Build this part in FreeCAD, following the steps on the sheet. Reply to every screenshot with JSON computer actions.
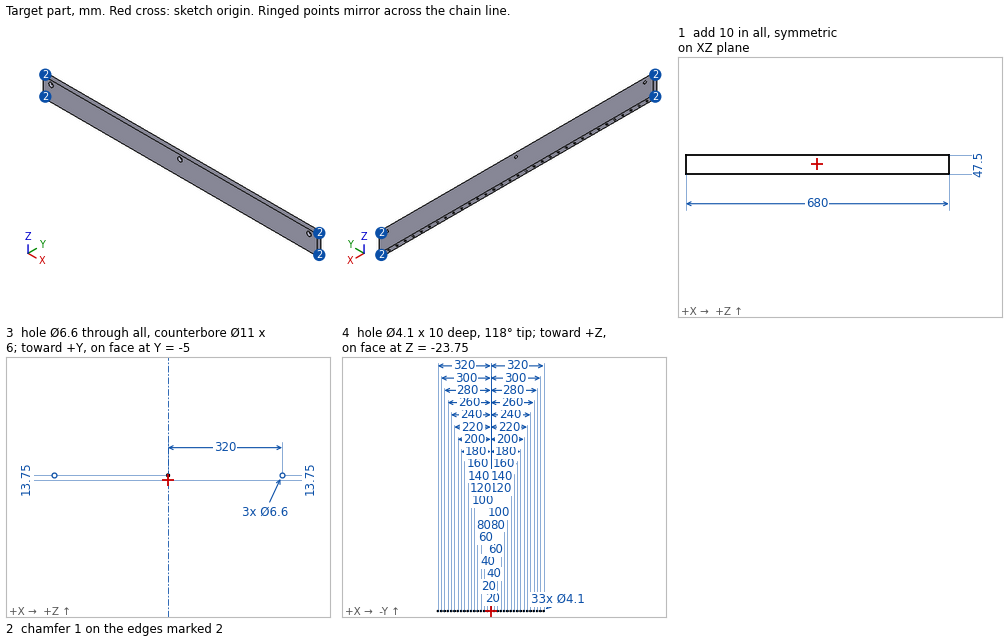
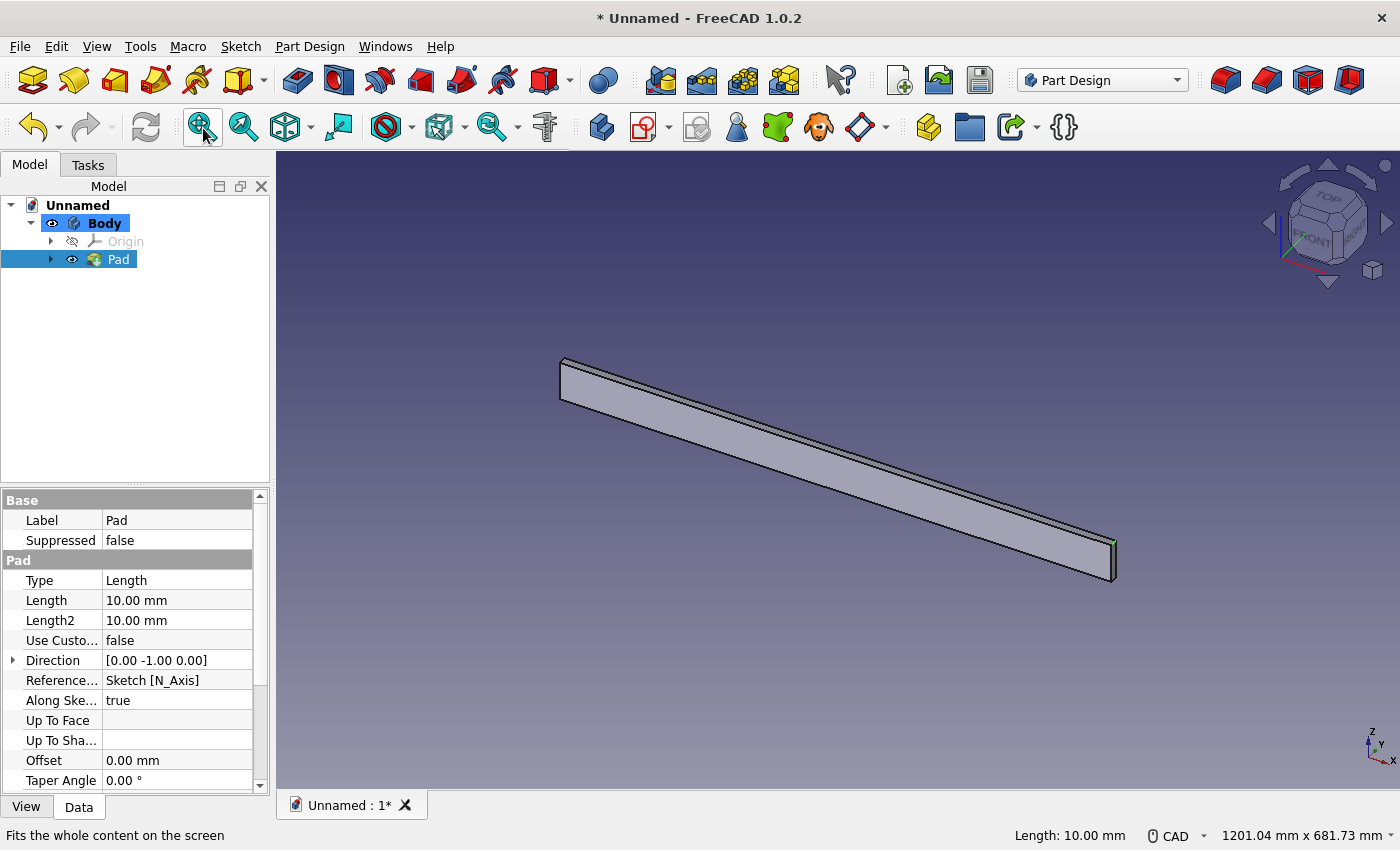
{"action": "key", "text": "0"}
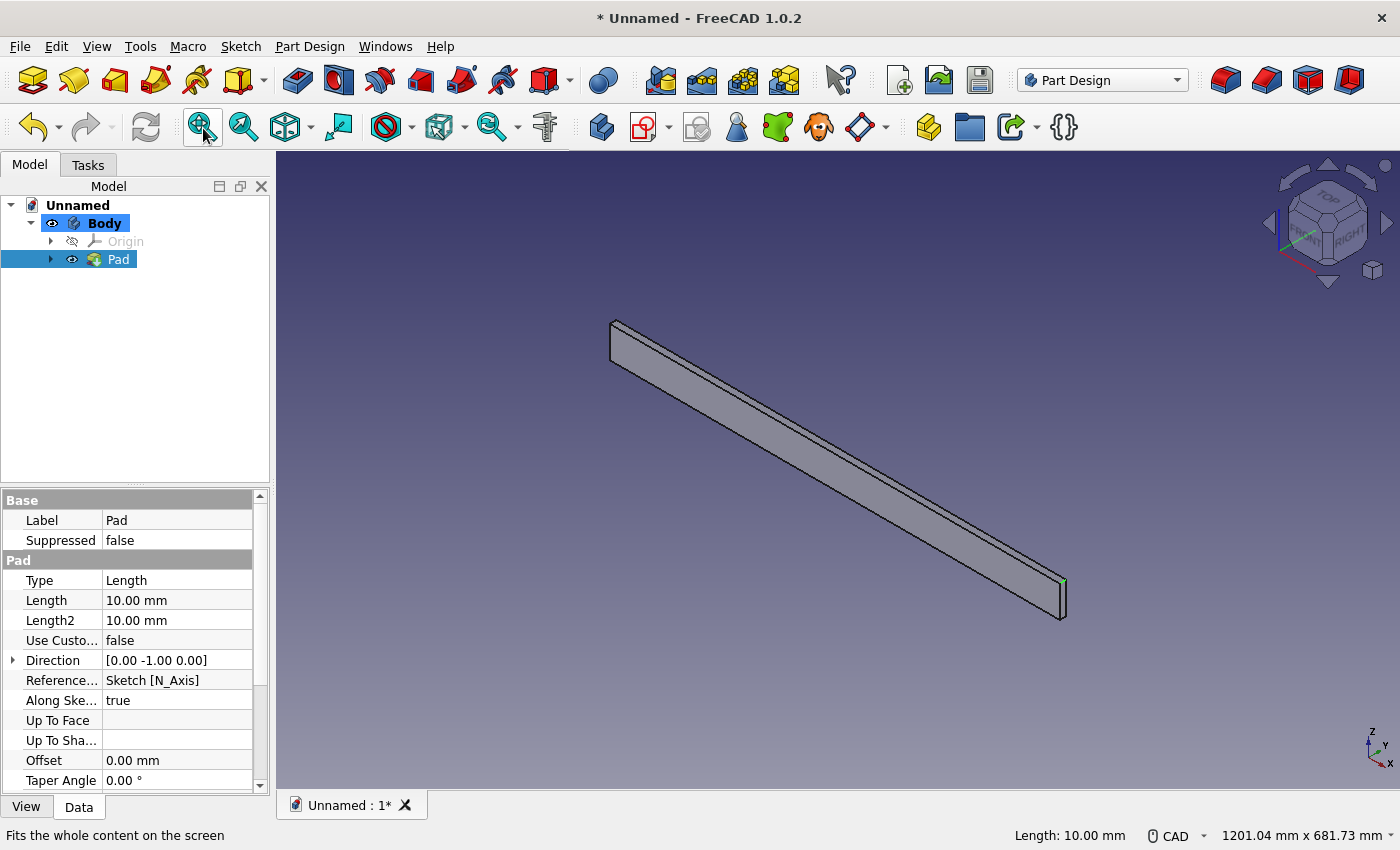
{"action": "scroll", "coordinate": [613, 321], "scroll_direction": "up", "scroll_amount": 8}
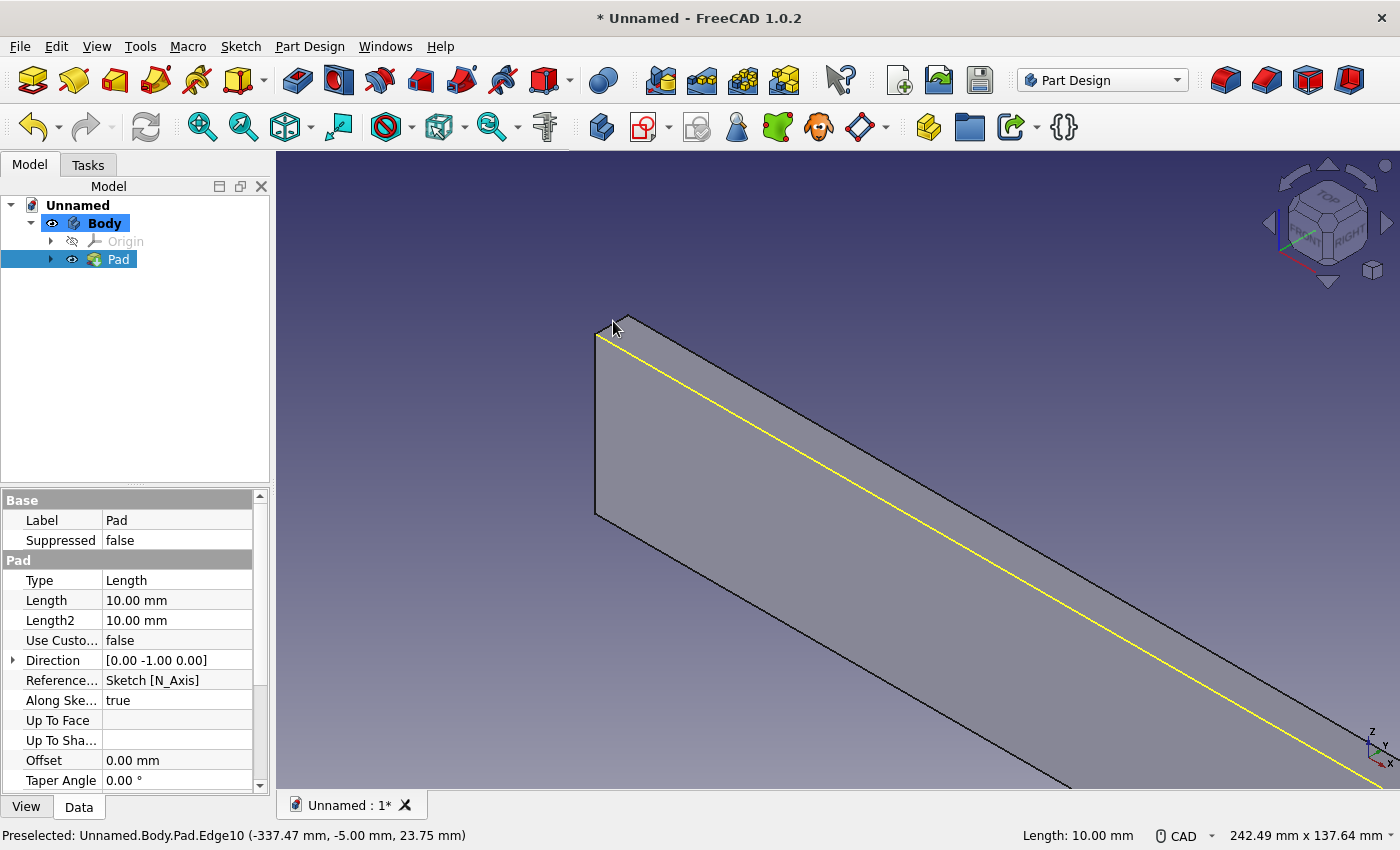
{"action": "left_click", "coordinate": [203, 128]}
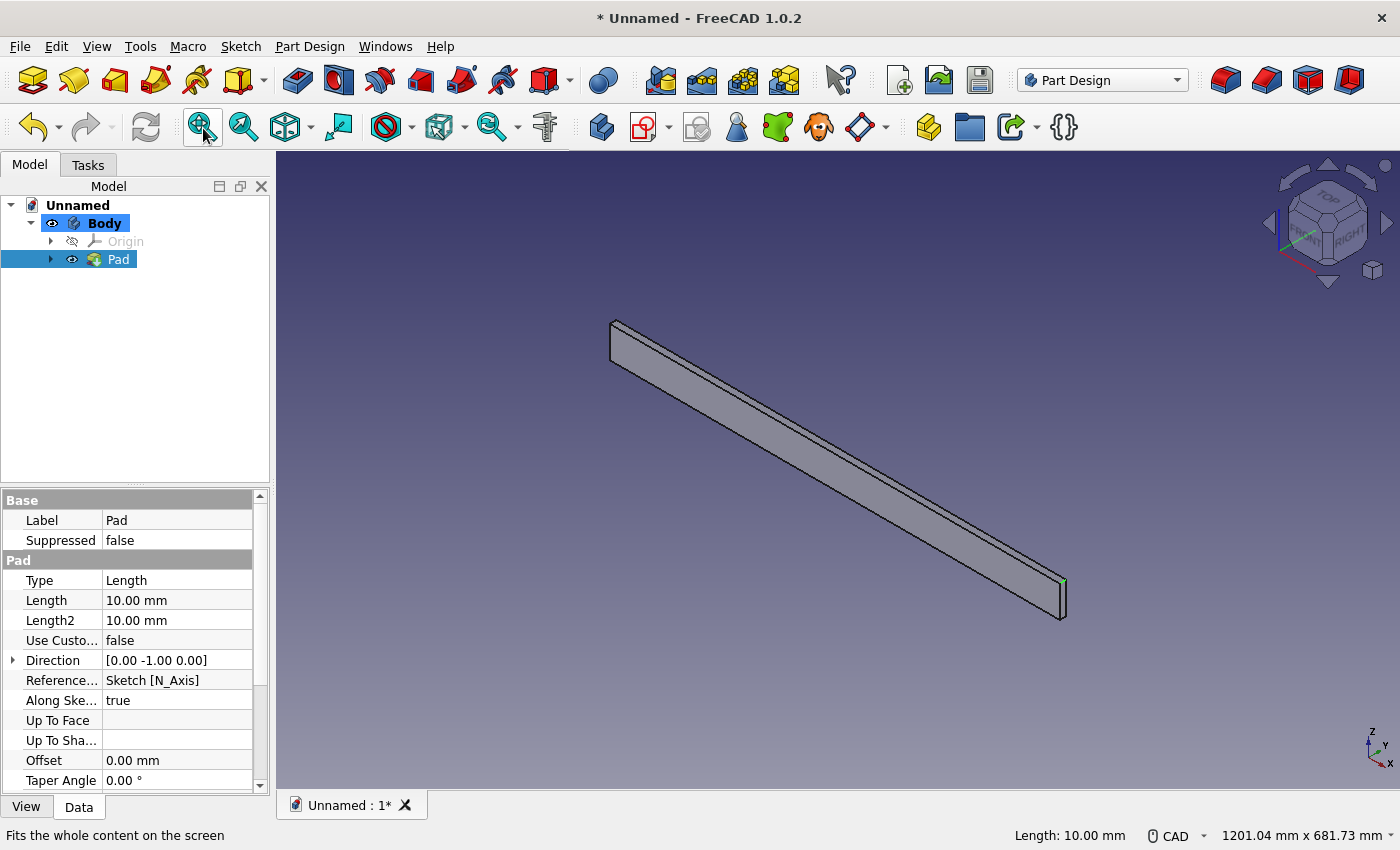
{"action": "key", "text": "2"}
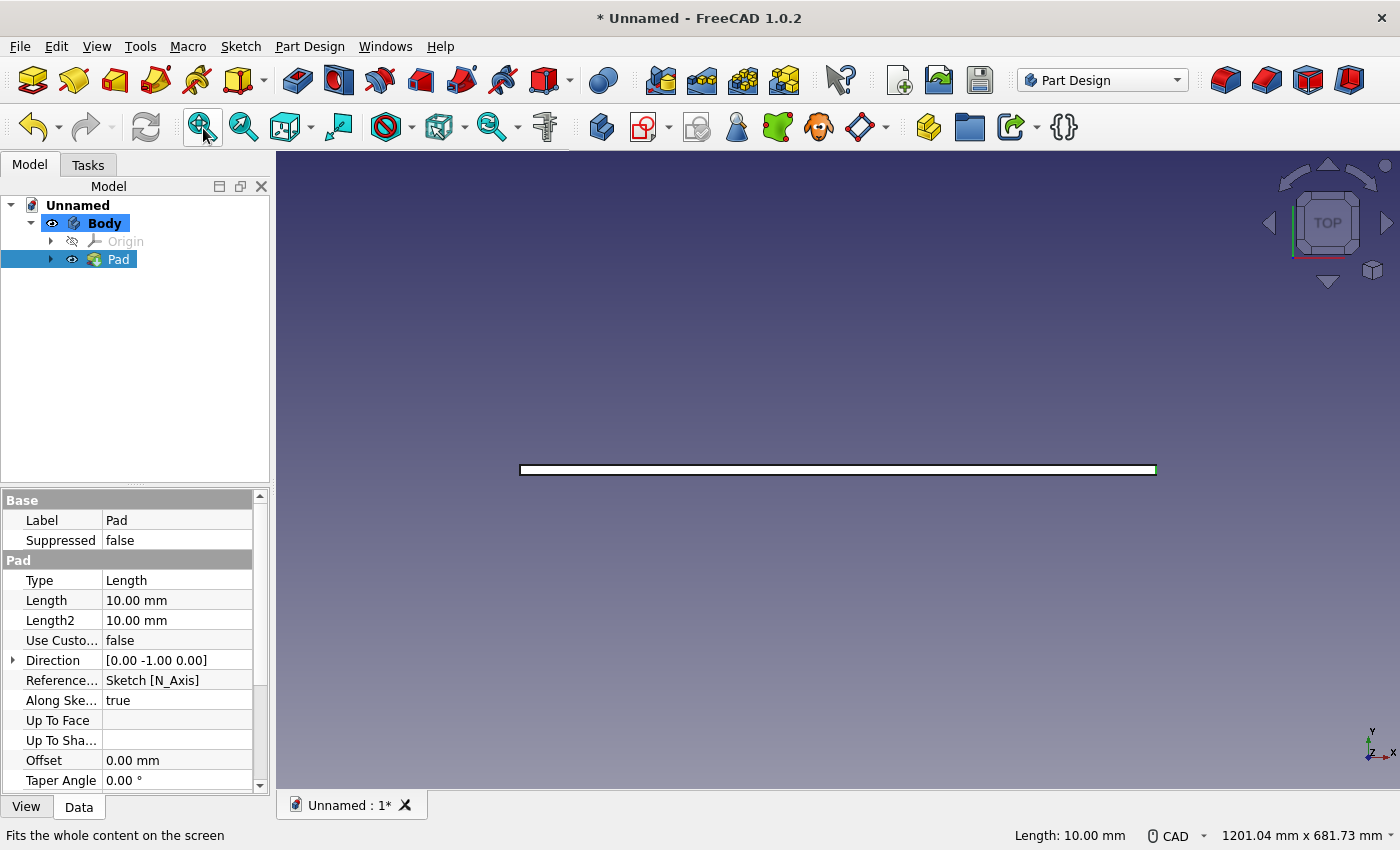
{"action": "left_click", "coordinate": [520, 471], "text": "ctrl"}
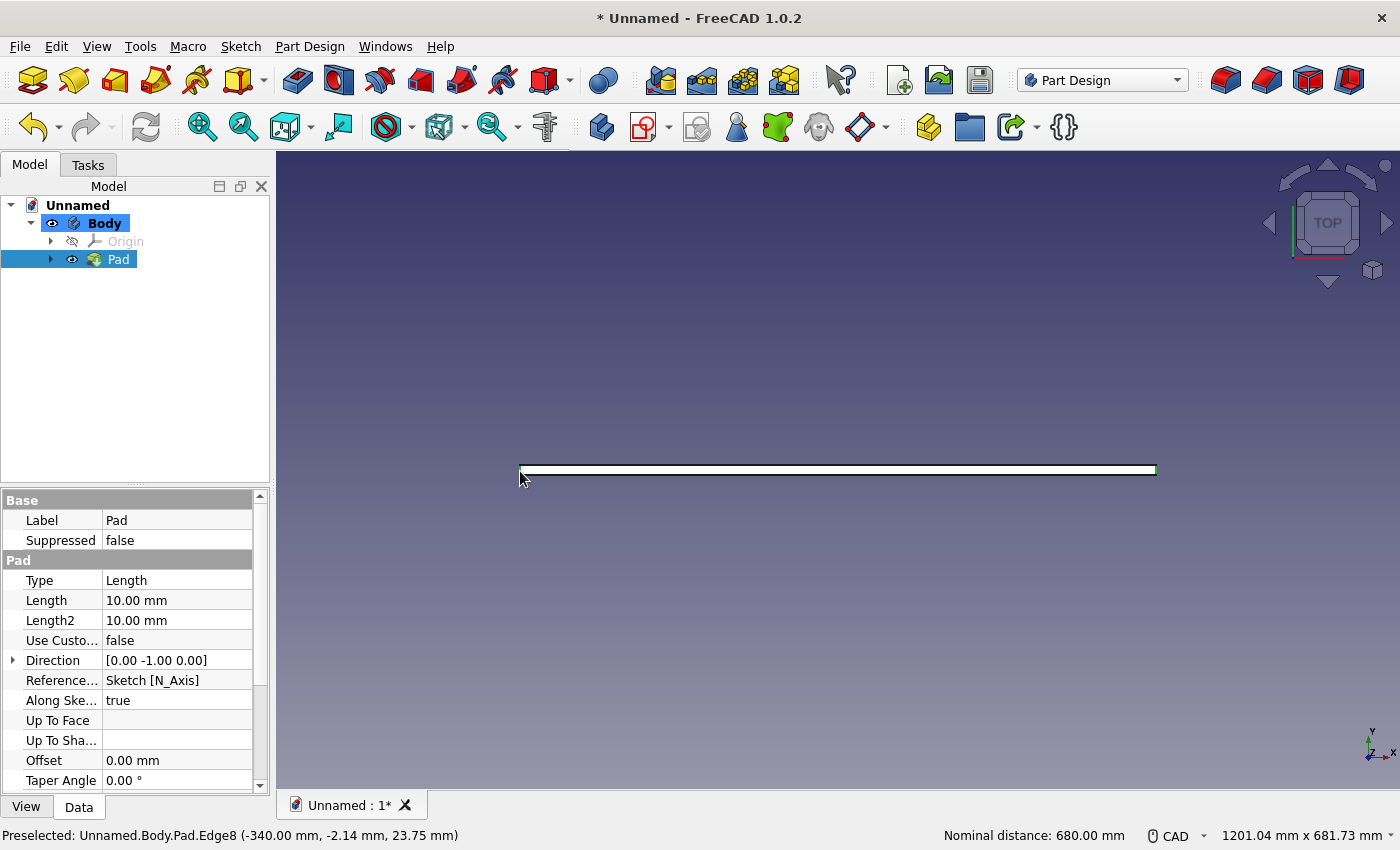
{"action": "scroll", "coordinate": [520, 469], "scroll_direction": "up", "scroll_amount": 8}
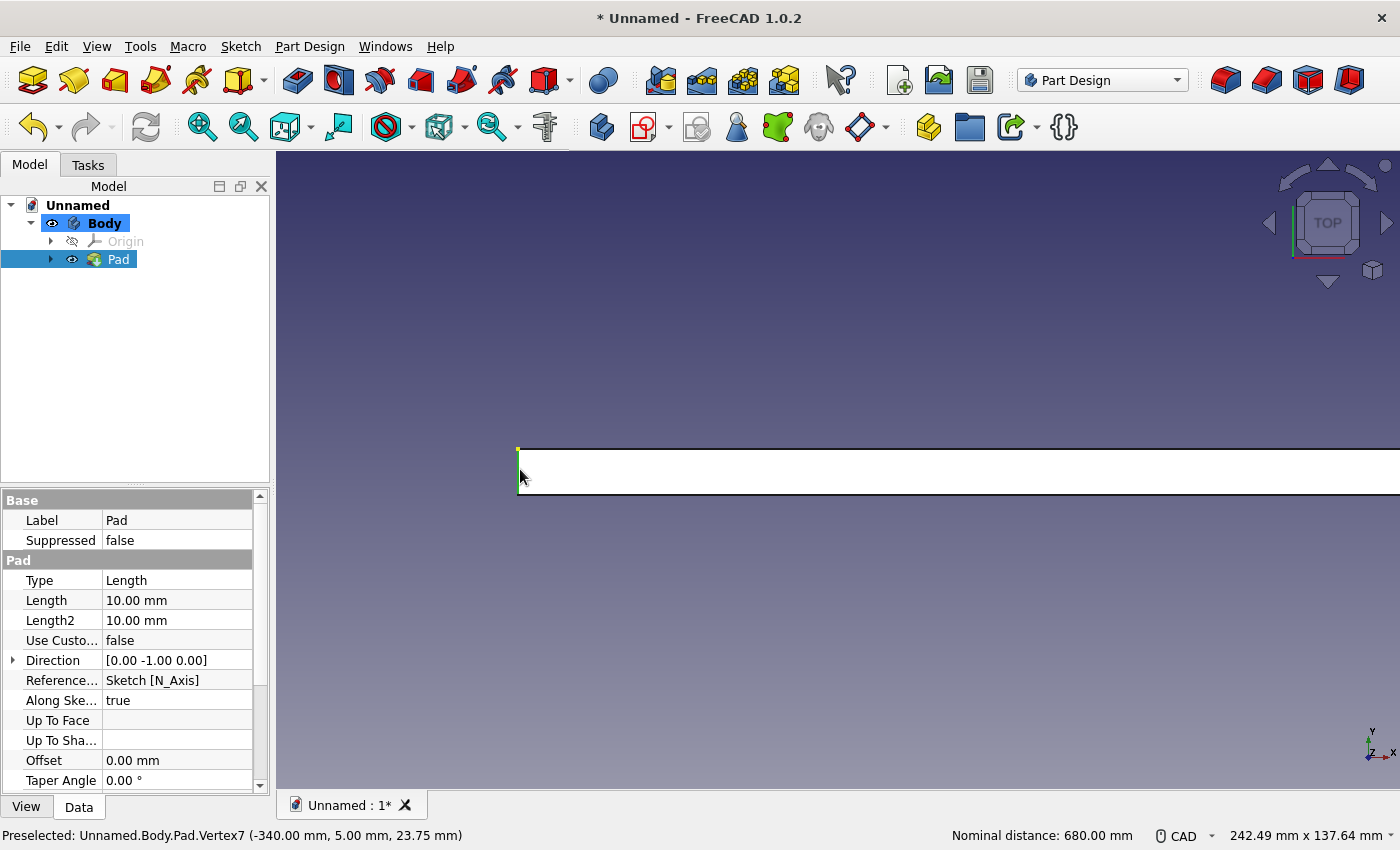
{"action": "left_click", "coordinate": [203, 128]}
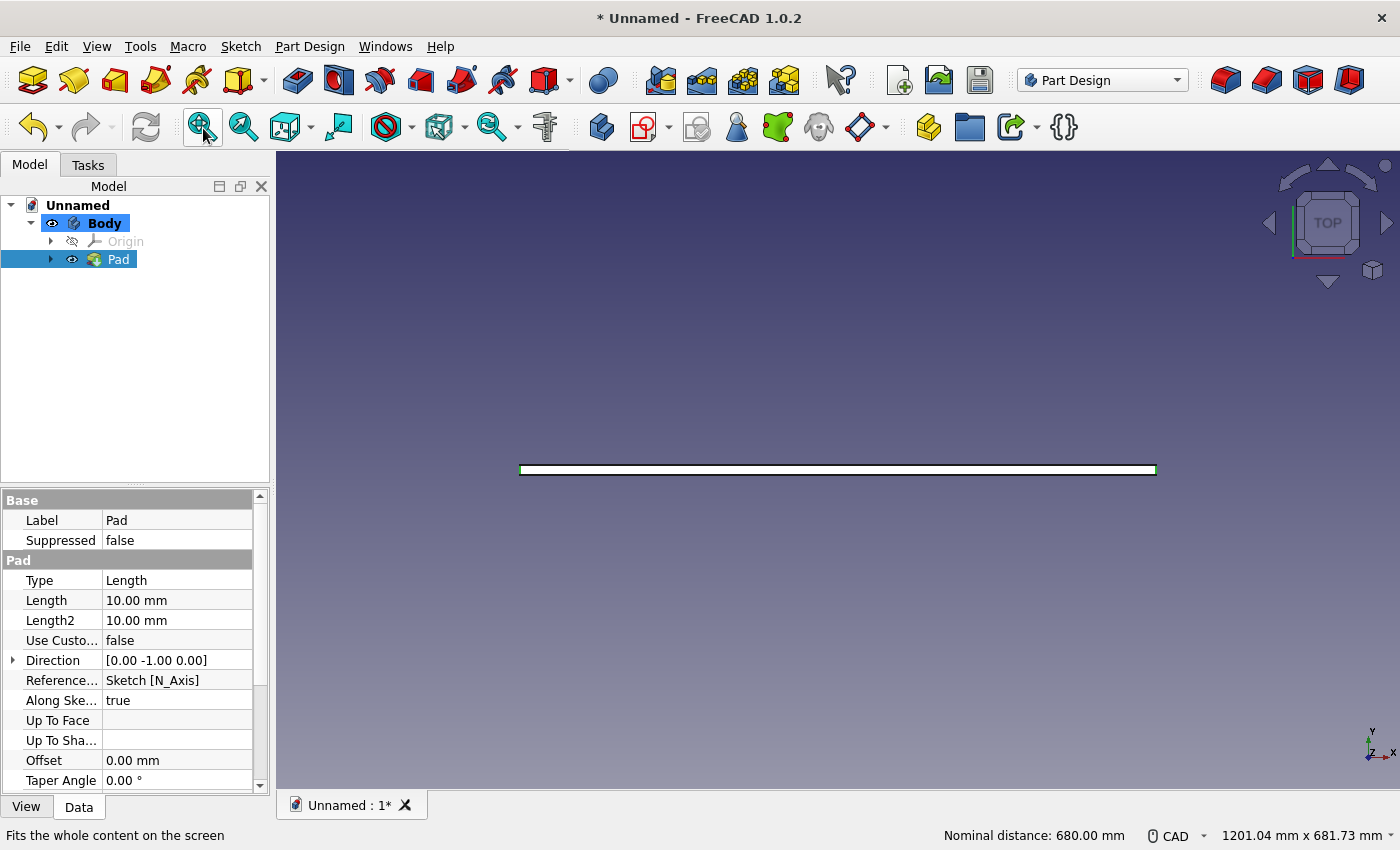
{"action": "key", "text": "1"}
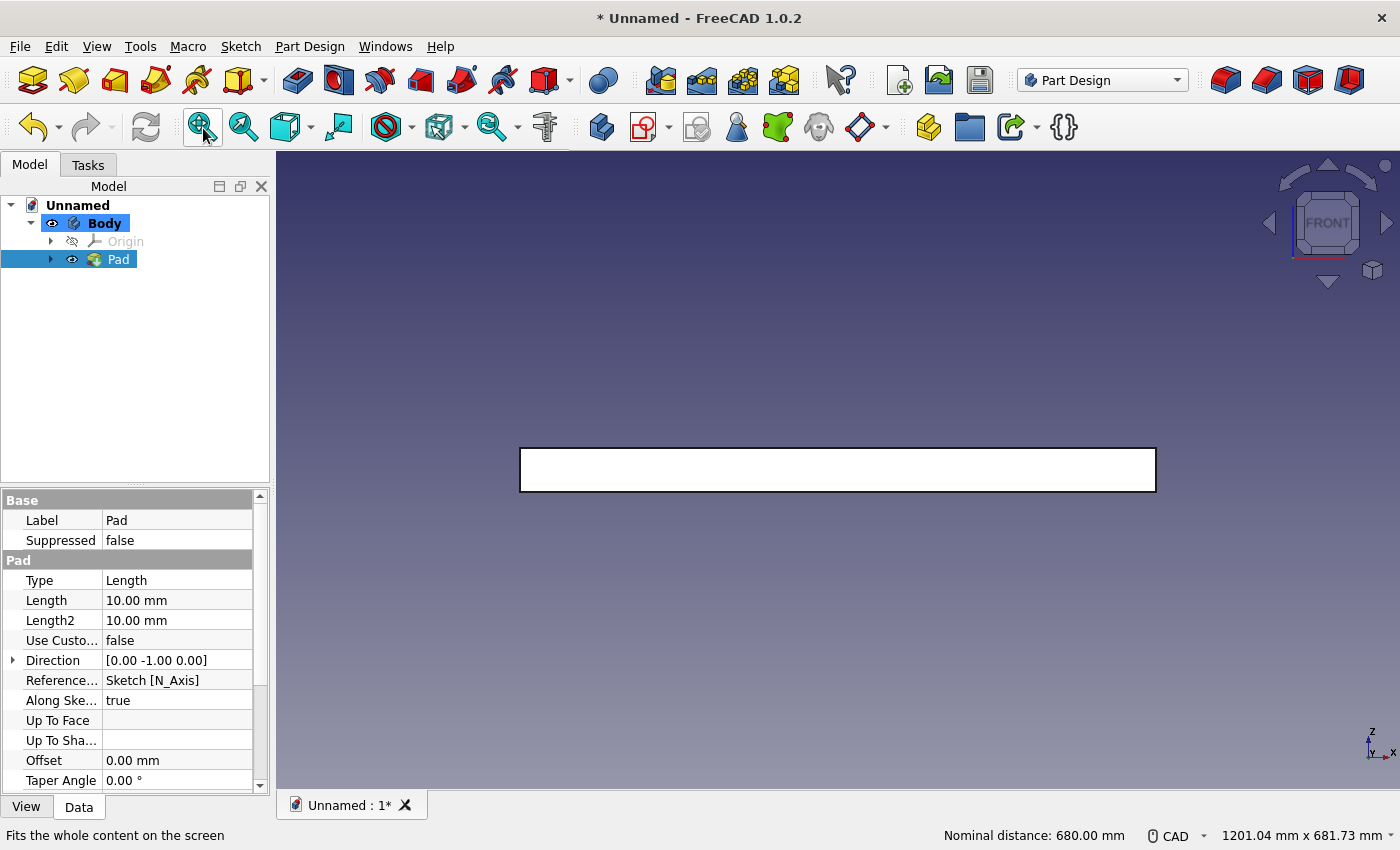
{"action": "scroll", "coordinate": [520, 491], "scroll_direction": "up", "scroll_amount": 8}